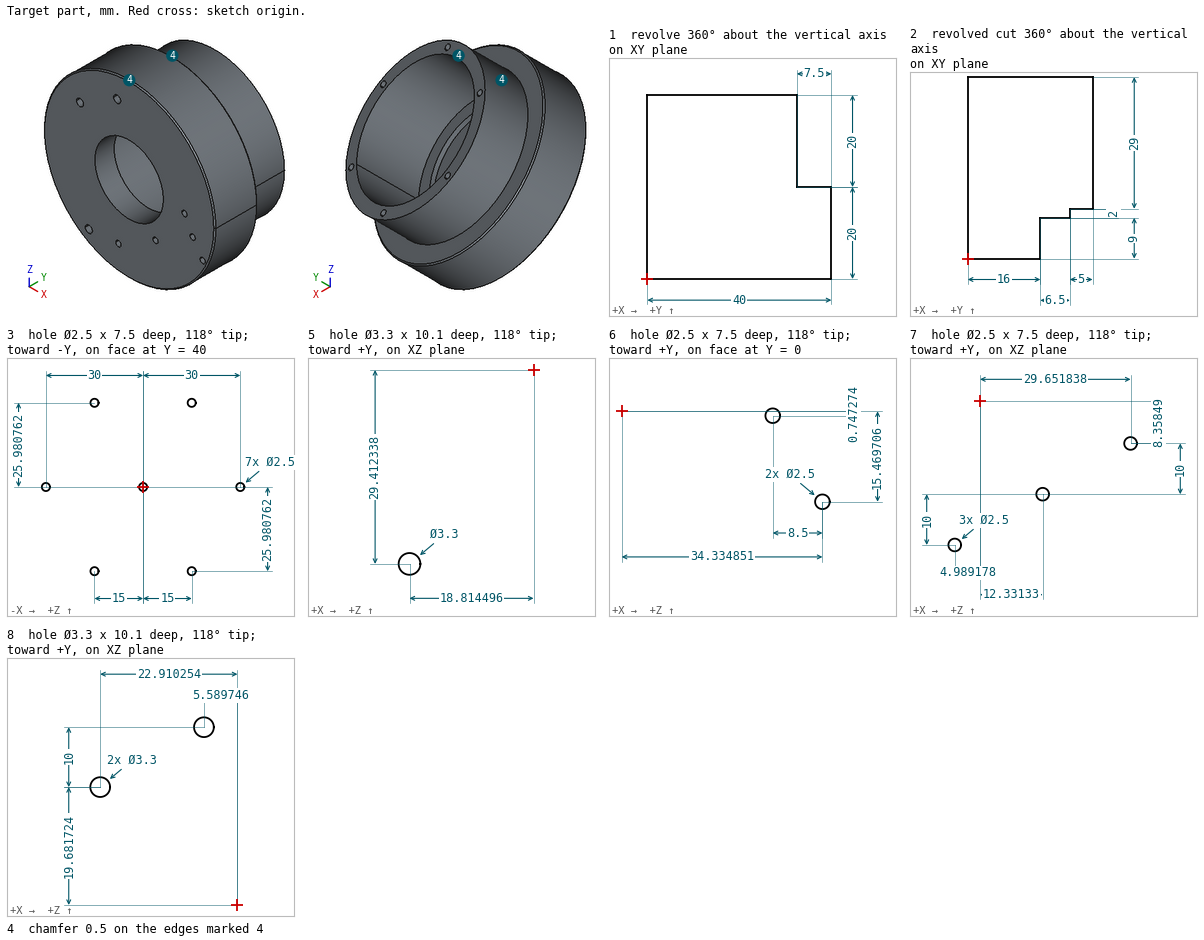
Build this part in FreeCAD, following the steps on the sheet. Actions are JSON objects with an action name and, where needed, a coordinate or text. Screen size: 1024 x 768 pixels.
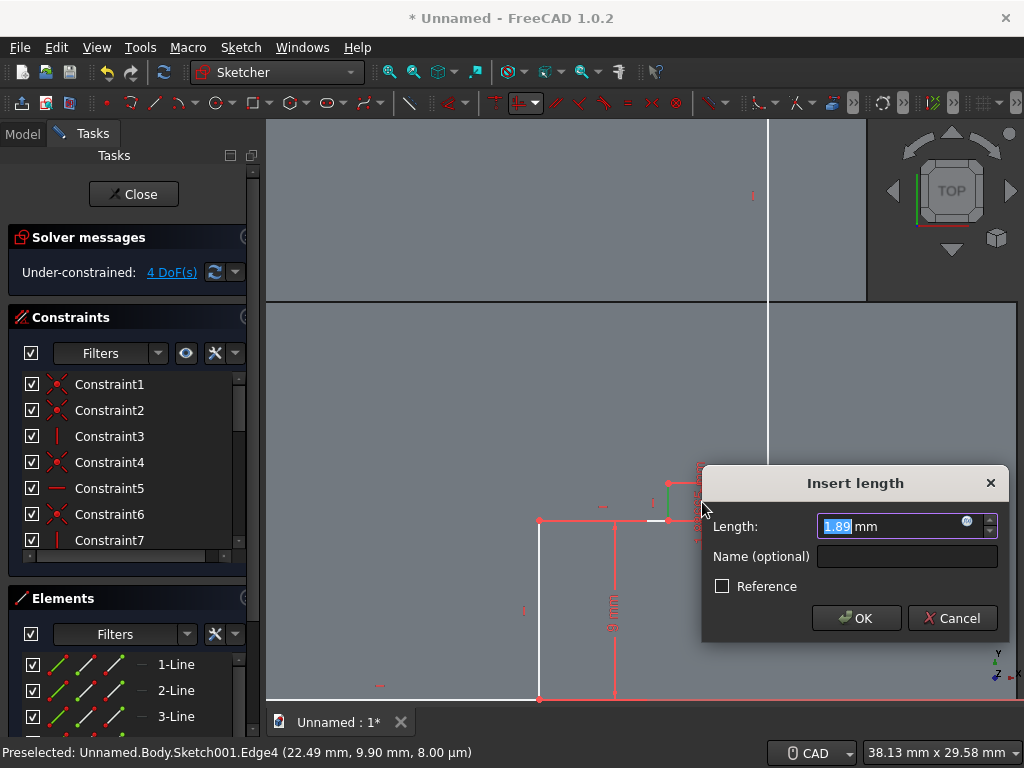
{"action": "type", "text": "2"}
{"action": "key", "text": "Return"}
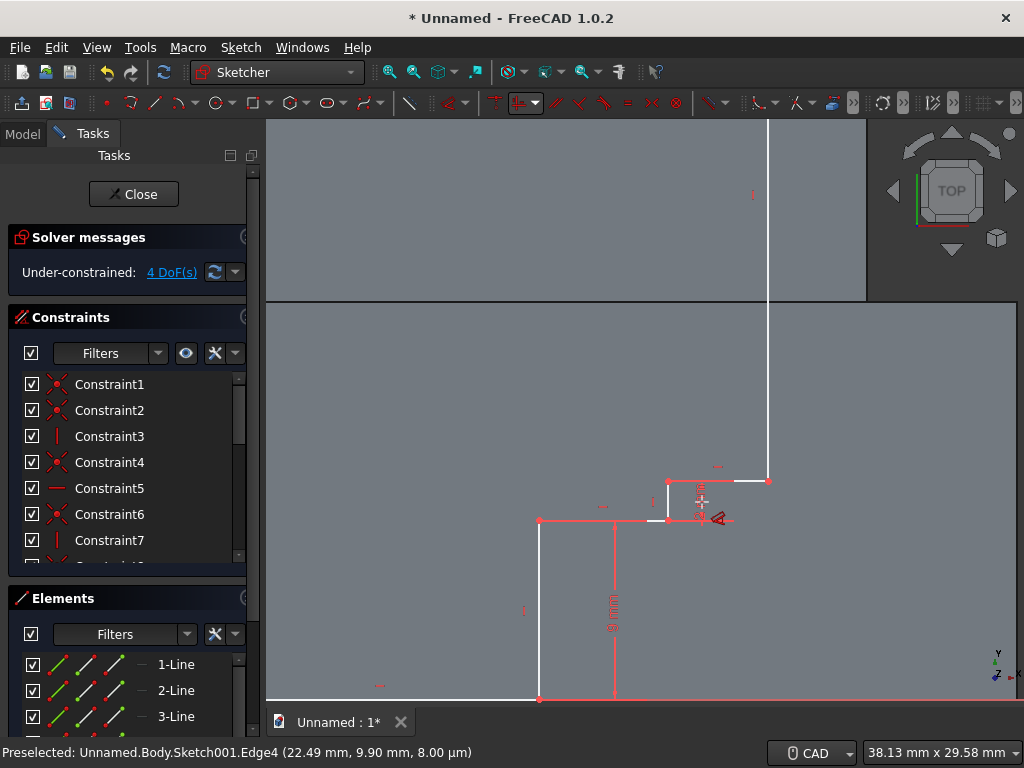
{"action": "left_click", "coordinate": [698, 481]}
{"action": "left_click", "coordinate": [718, 447]}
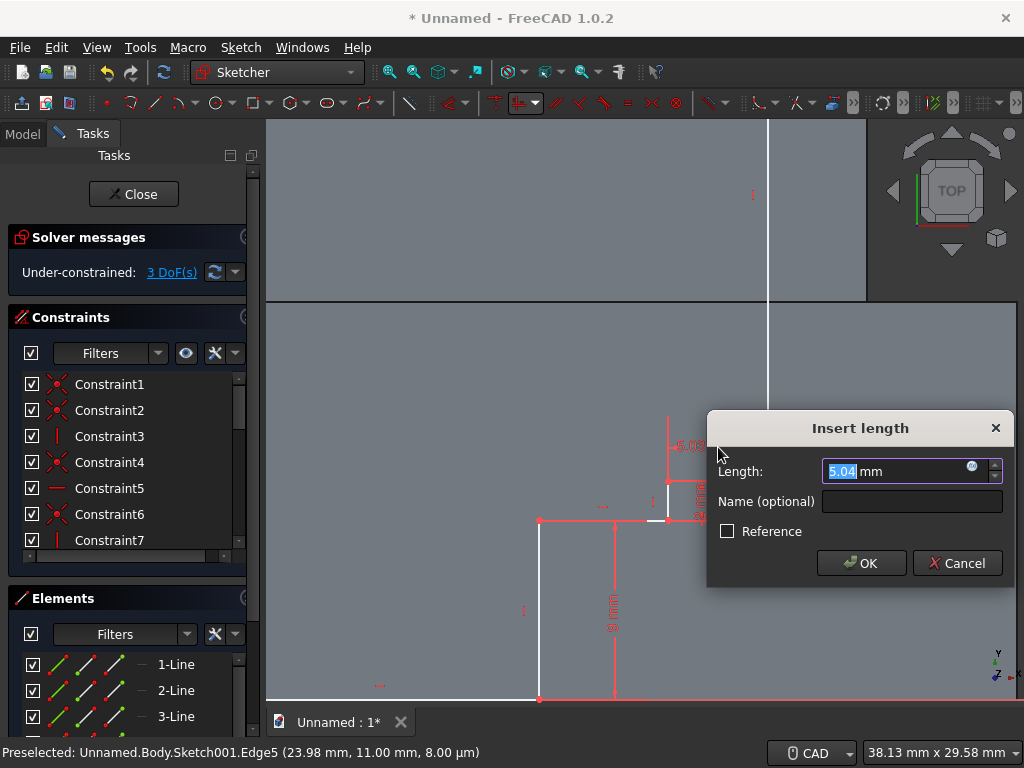
{"action": "type", "text": "5"}
{"action": "key", "text": "Return"}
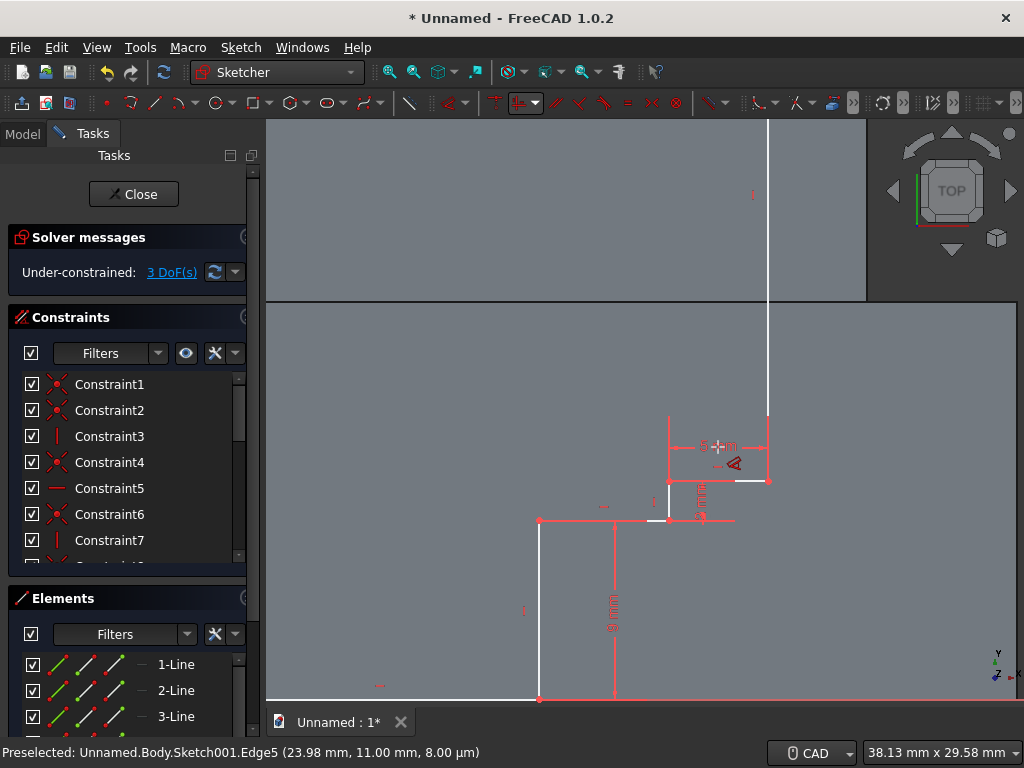
{"action": "scroll", "coordinate": [643, 503], "scroll_direction": "down", "scroll_amount": 4}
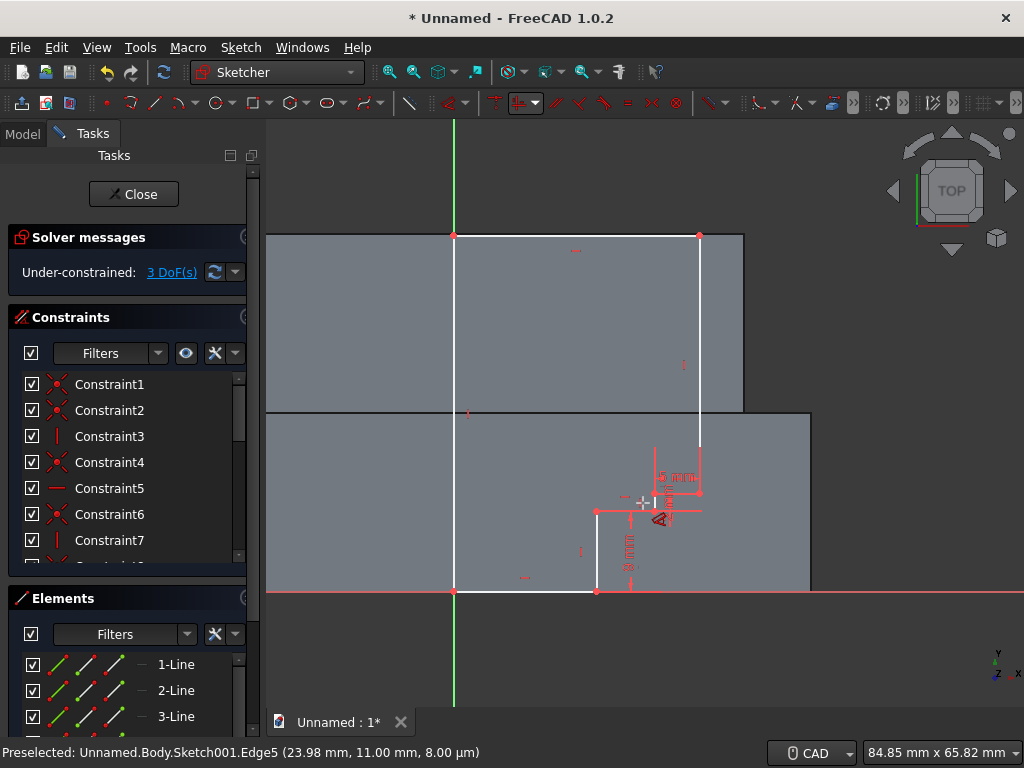
{"action": "left_click", "coordinate": [497, 592]}
{"action": "left_click", "coordinate": [525, 626]}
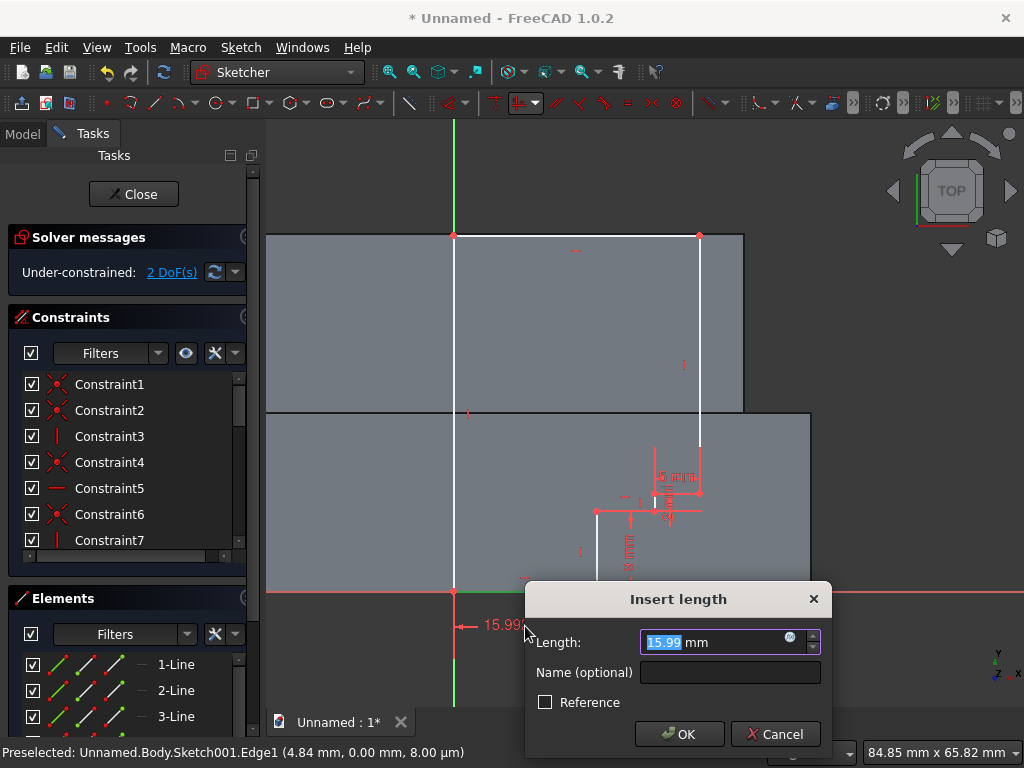
{"action": "type", "text": "16"}
{"action": "key", "text": "Return"}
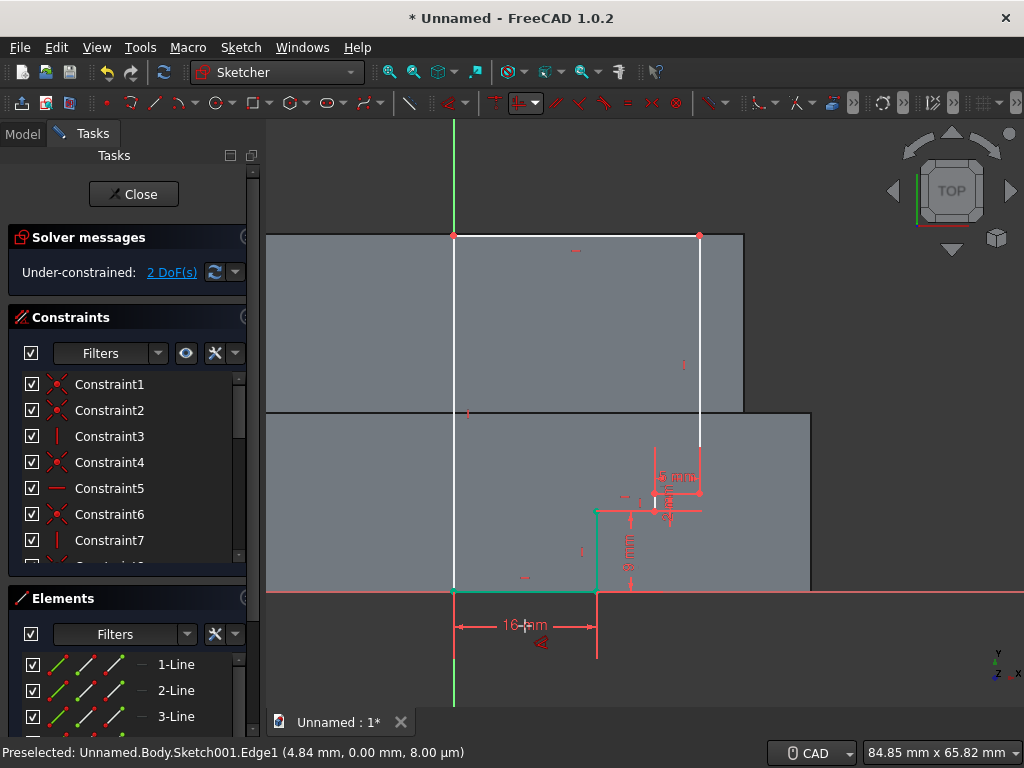
{"action": "left_click", "coordinate": [700, 416]}
{"action": "left_click", "coordinate": [734, 365]}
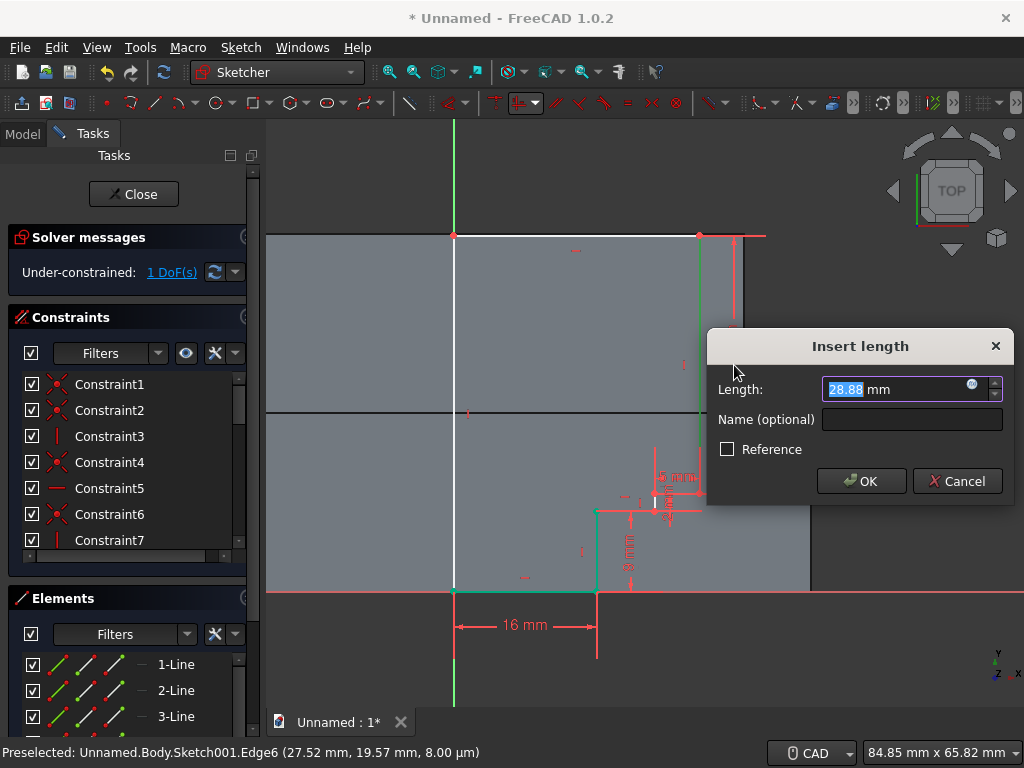
{"action": "type", "text": "29"}
{"action": "key", "text": "Return"}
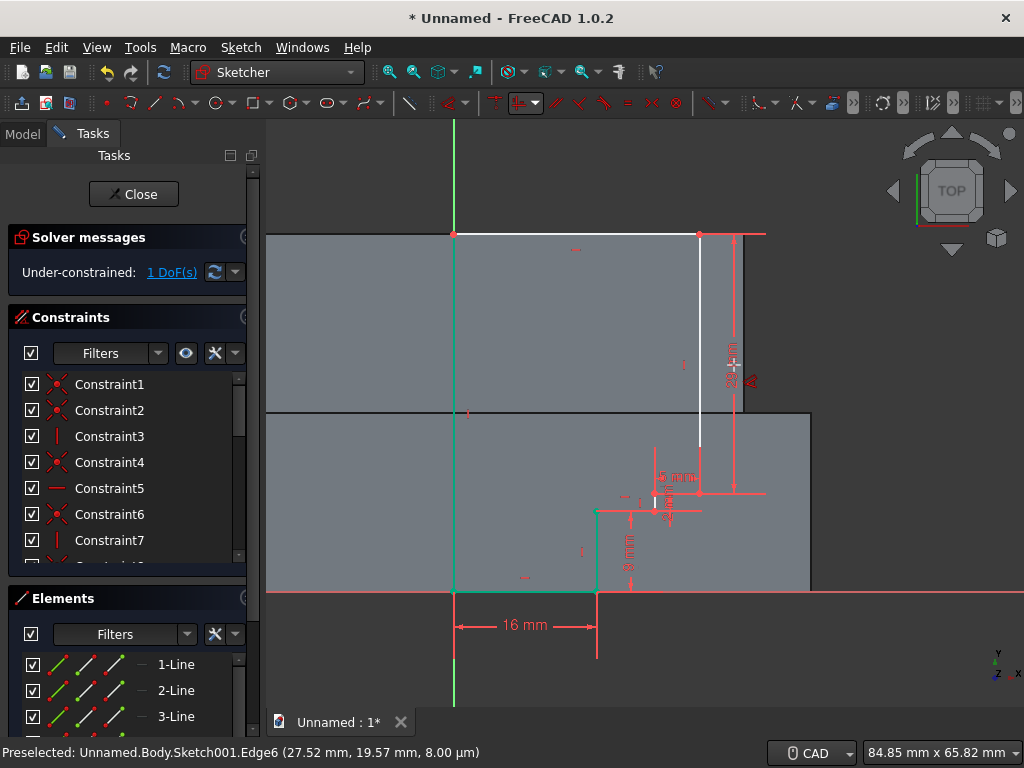
{"action": "left_click", "coordinate": [614, 511]}
{"action": "left_click", "coordinate": [605, 477]}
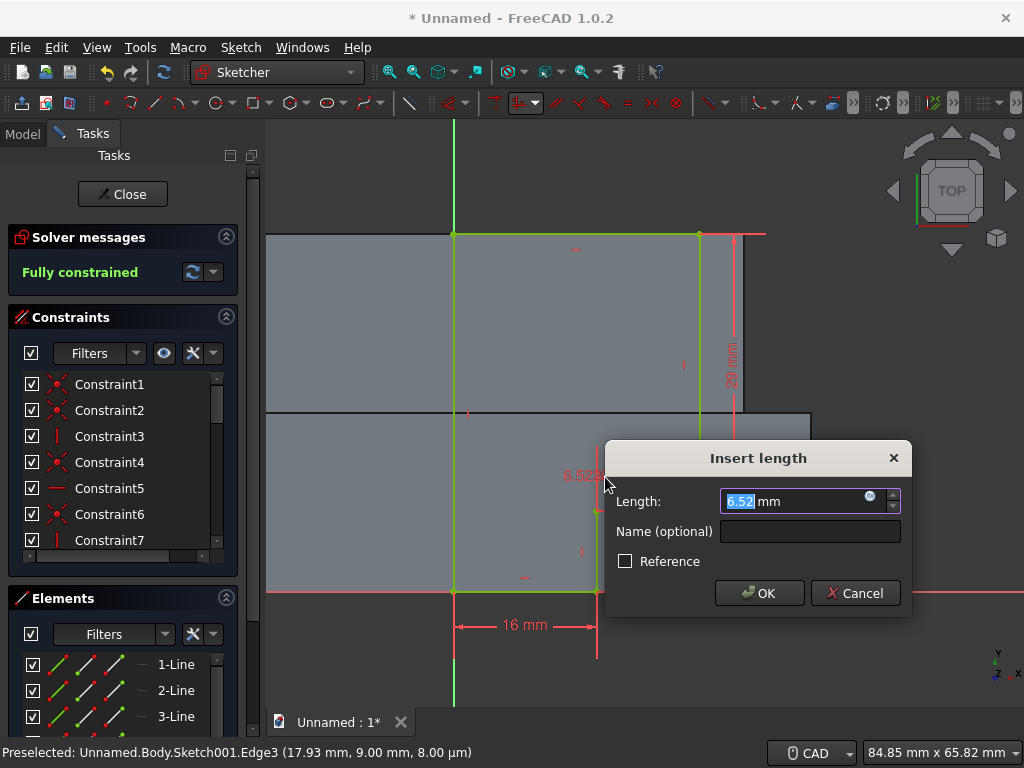
{"action": "type", "text": "6.5"}
{"action": "key", "text": "Return"}
{"action": "key", "text": "Escape"}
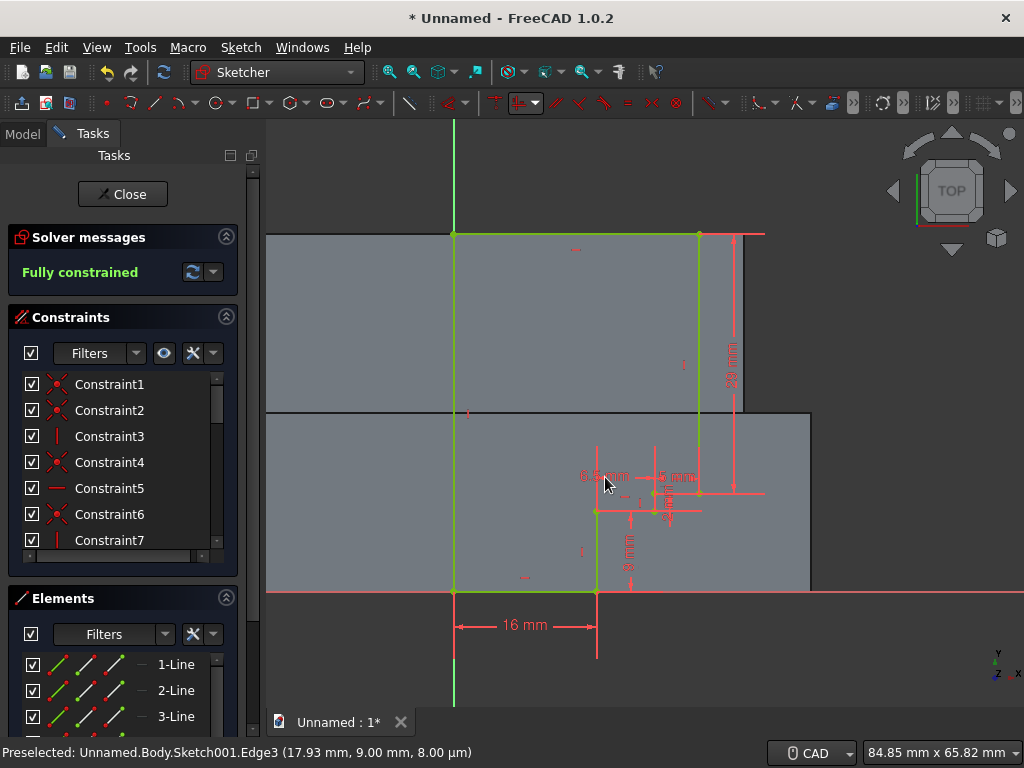
{"action": "left_click", "coordinate": [123, 194]}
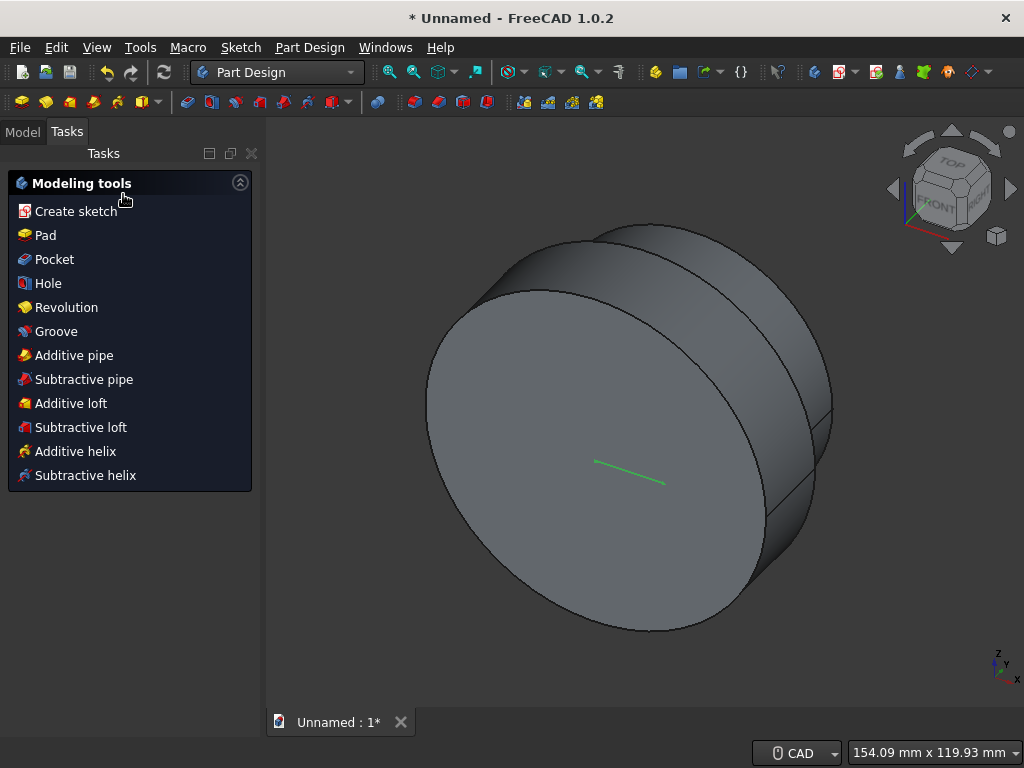
{"action": "left_click", "coordinate": [236, 102]}